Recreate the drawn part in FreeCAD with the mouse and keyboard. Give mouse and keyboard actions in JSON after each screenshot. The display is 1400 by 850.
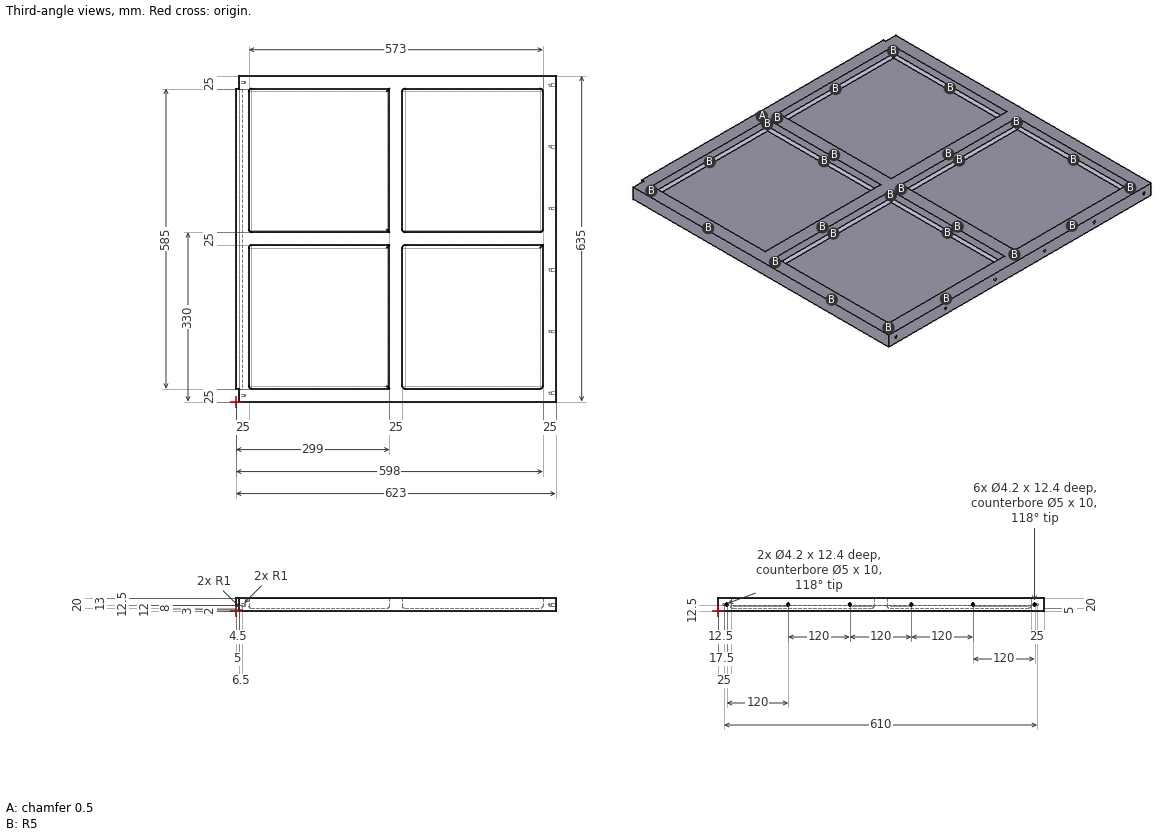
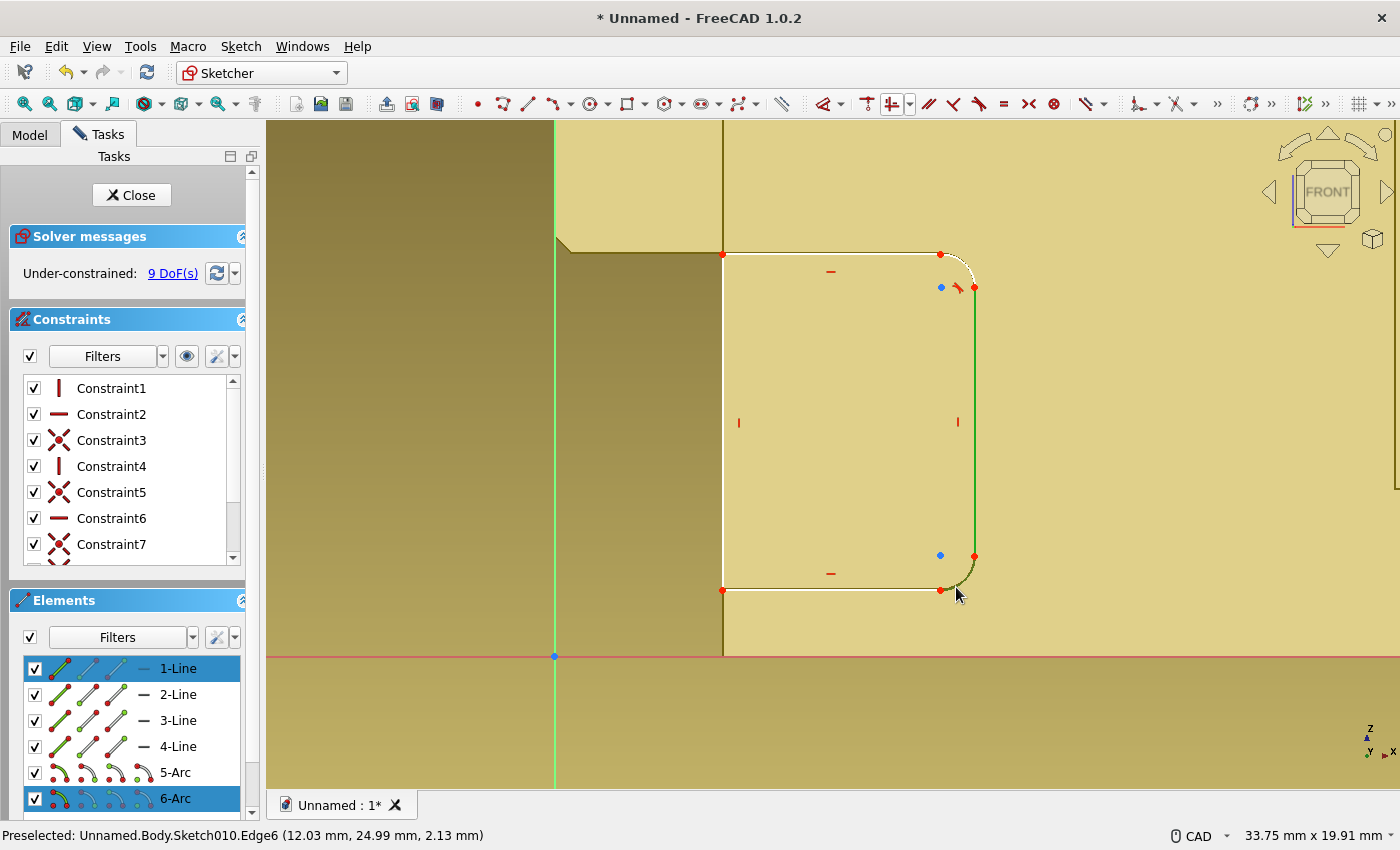
{"action": "left_click", "coordinate": [979, 104]}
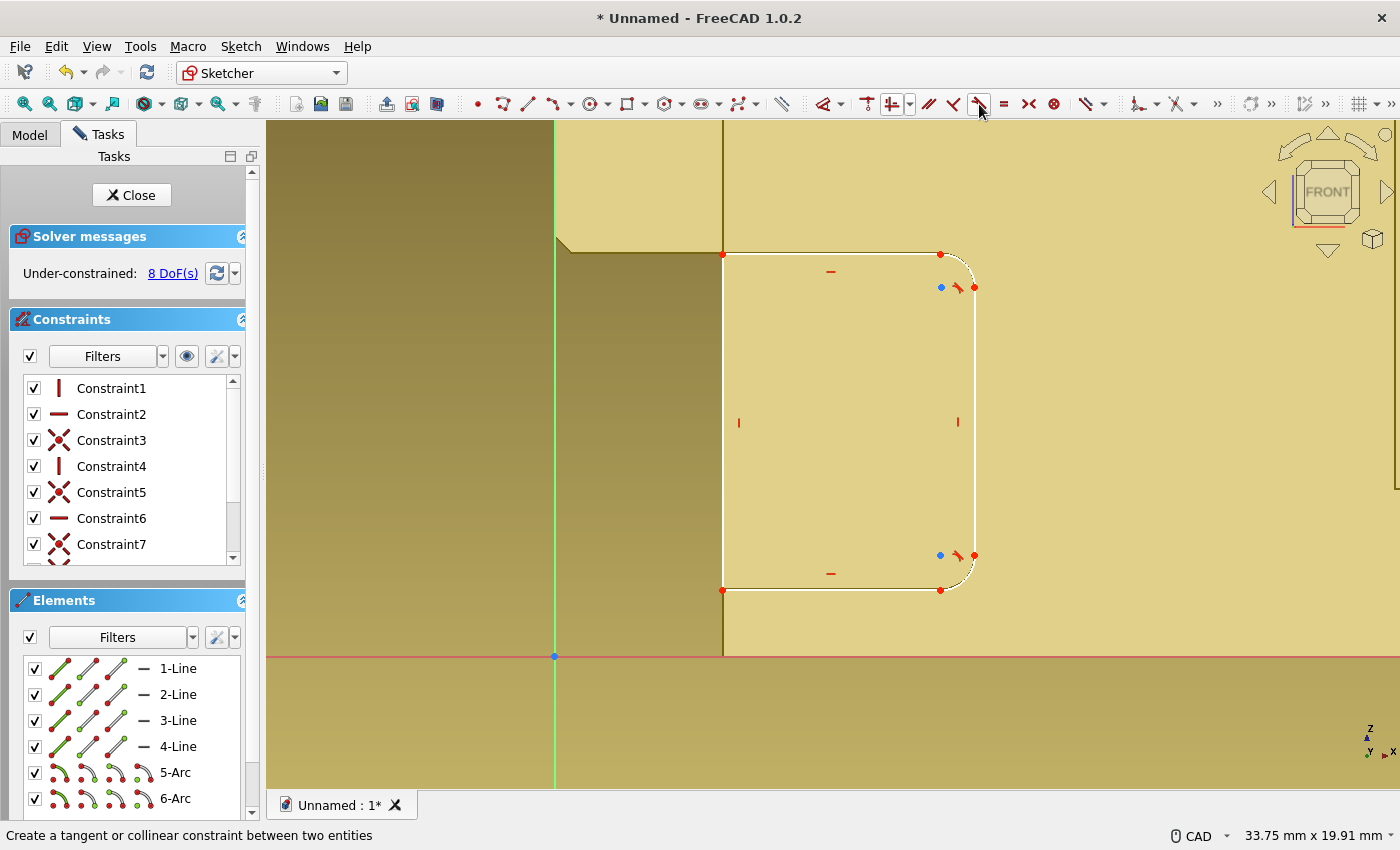
{"action": "left_click", "coordinate": [876, 254]}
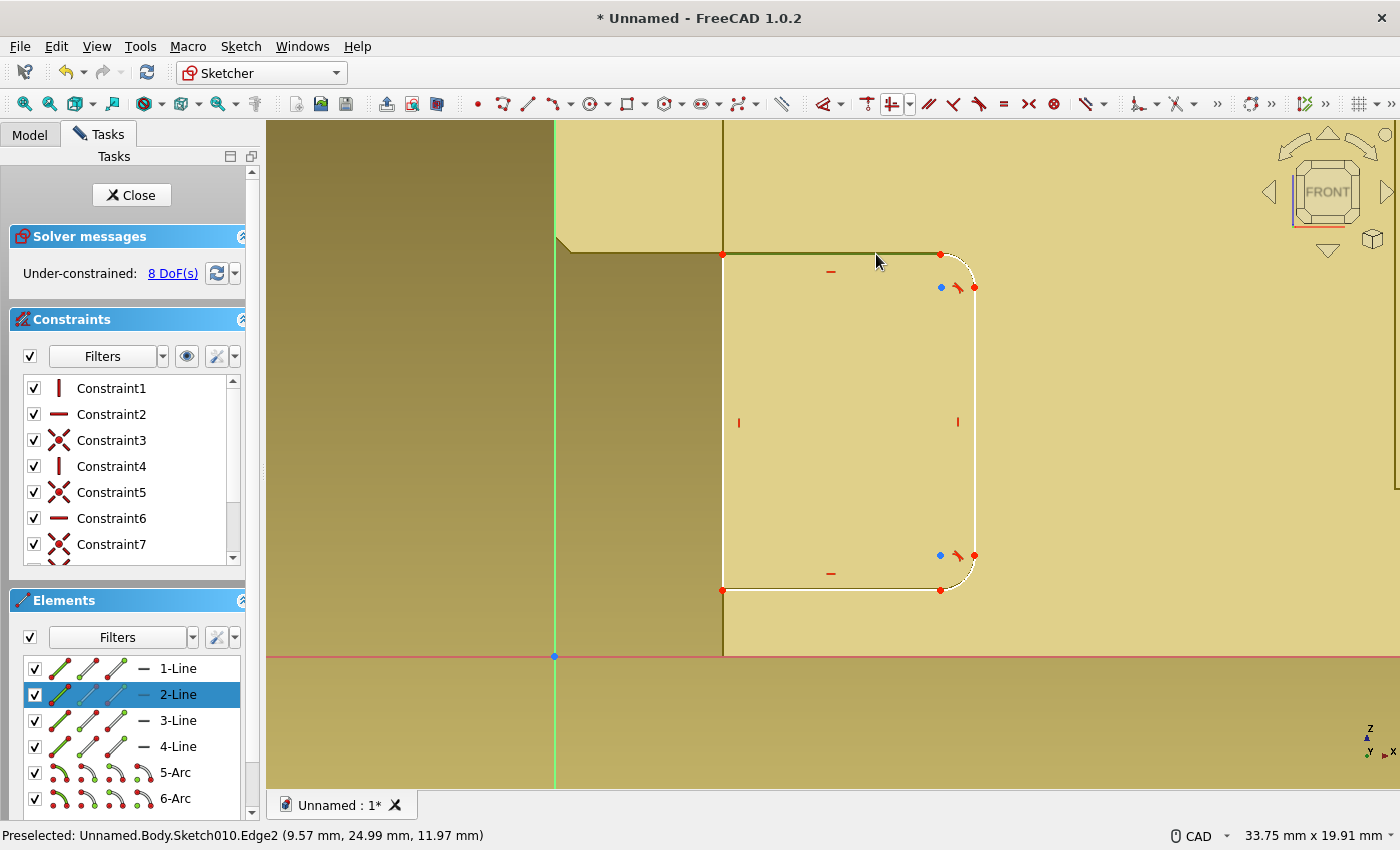
{"action": "left_click", "coordinate": [971, 272]}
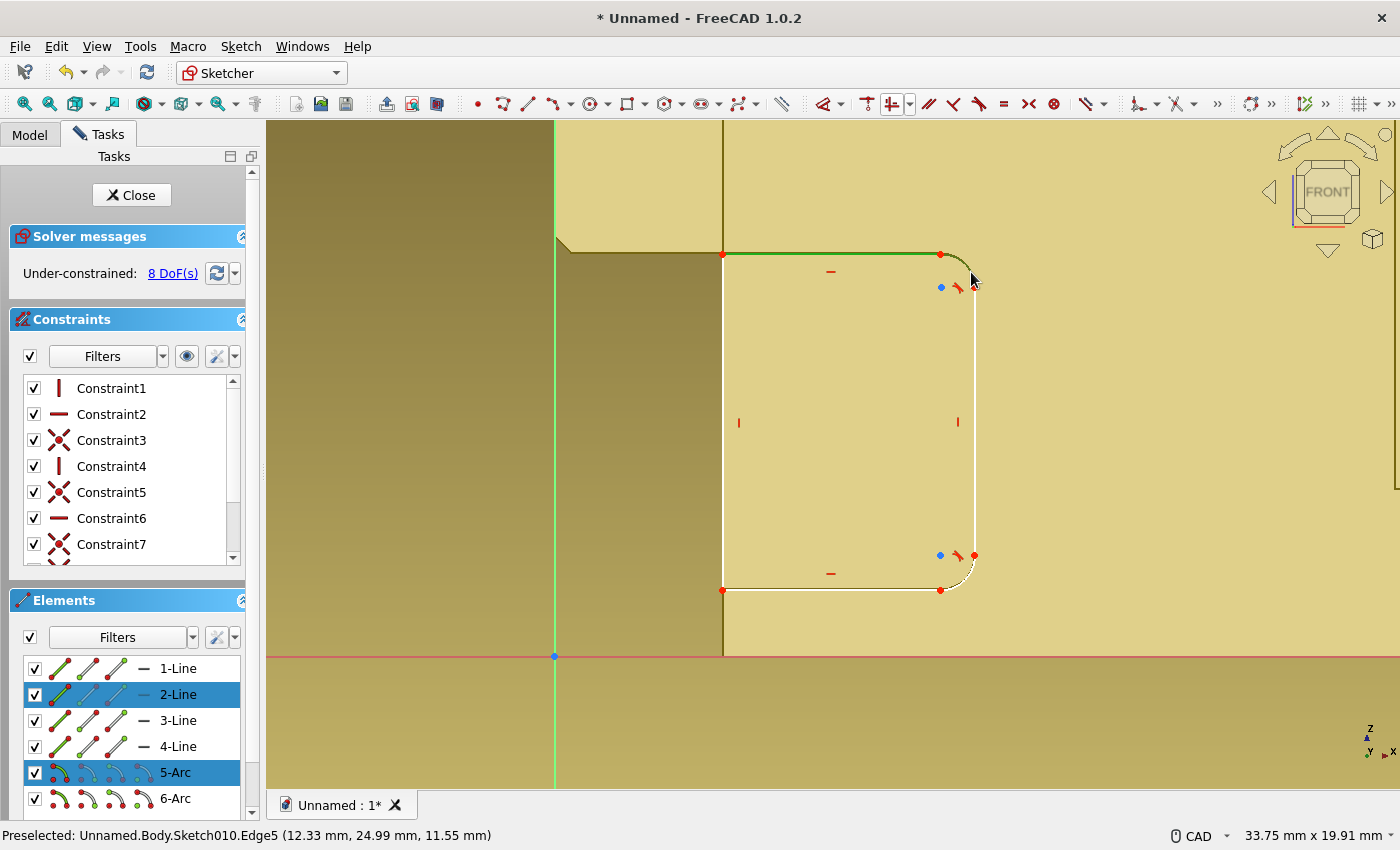
{"action": "key", "text": "t"}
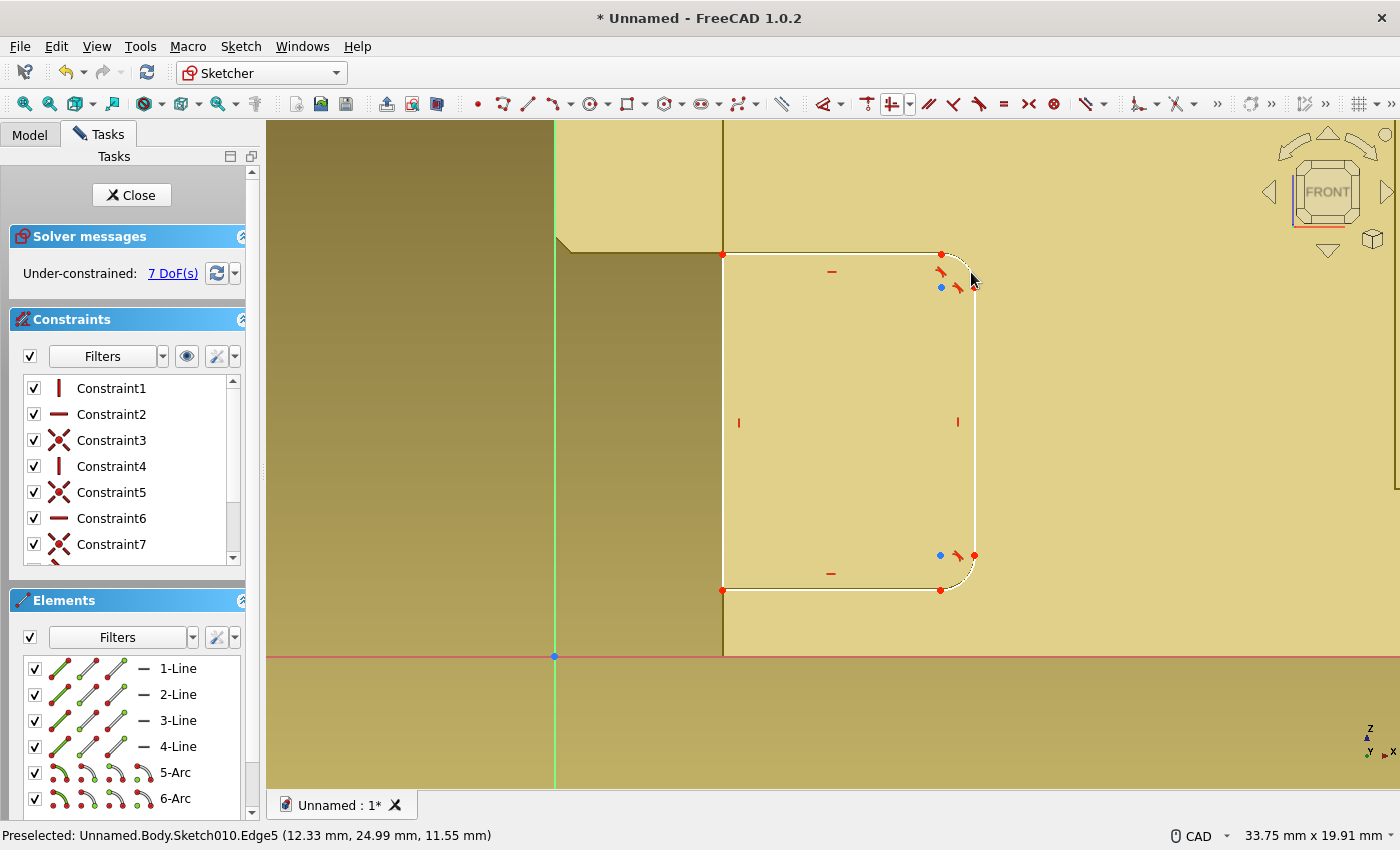
{"action": "left_click", "coordinate": [788, 590]}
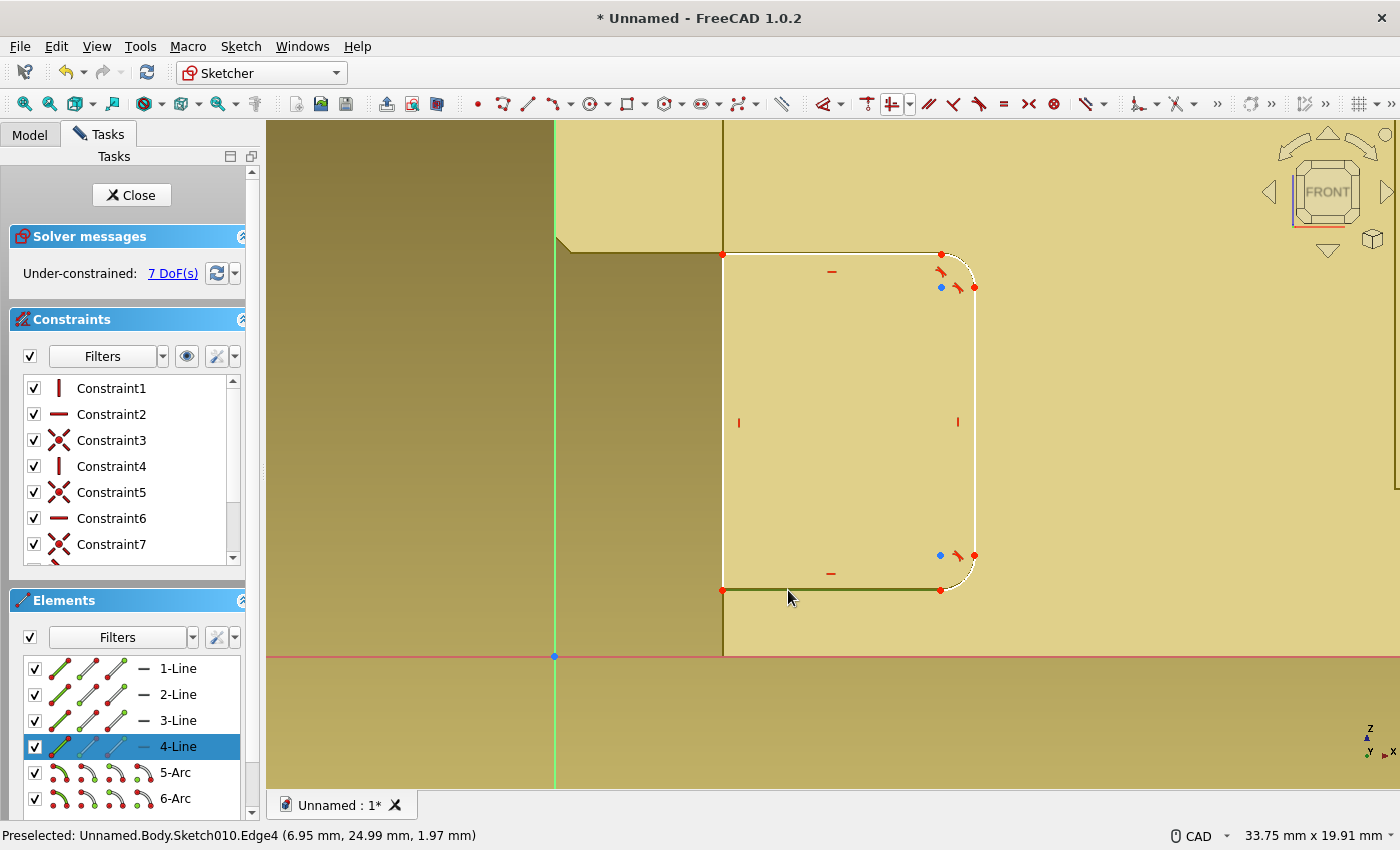
{"action": "left_click", "coordinate": [956, 586]}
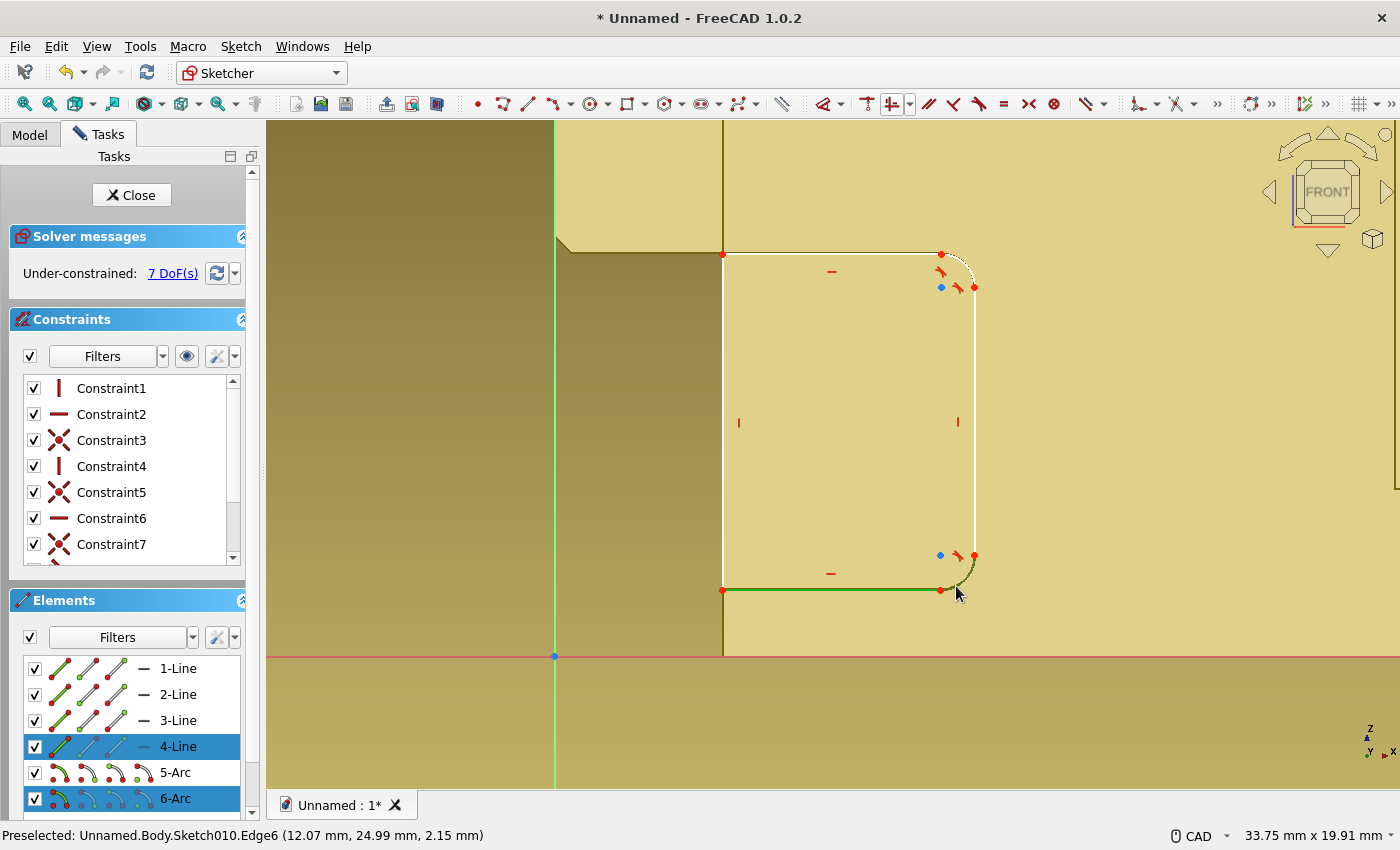
{"action": "left_click", "coordinate": [979, 104]}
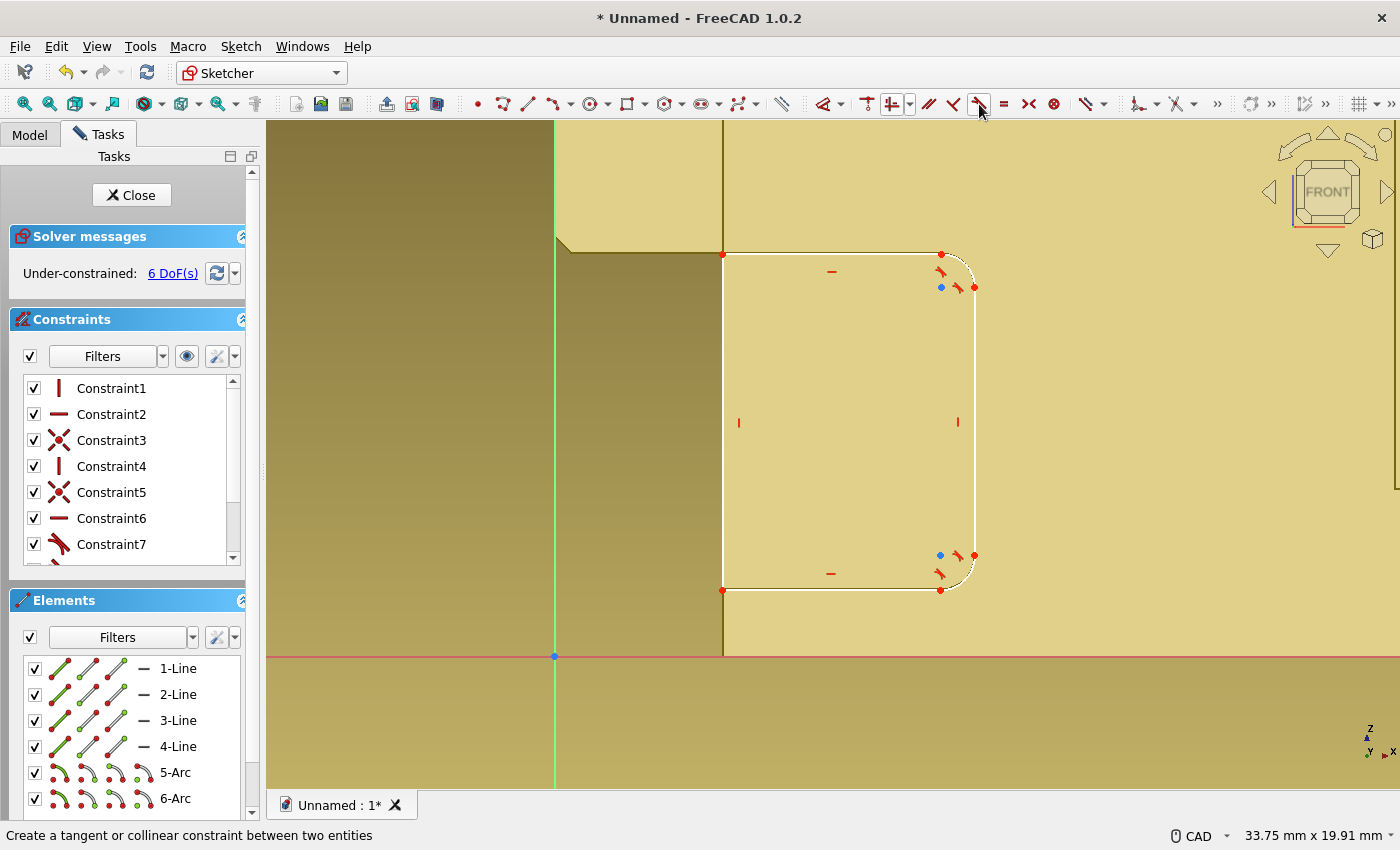
{"action": "left_click", "coordinate": [971, 272]}